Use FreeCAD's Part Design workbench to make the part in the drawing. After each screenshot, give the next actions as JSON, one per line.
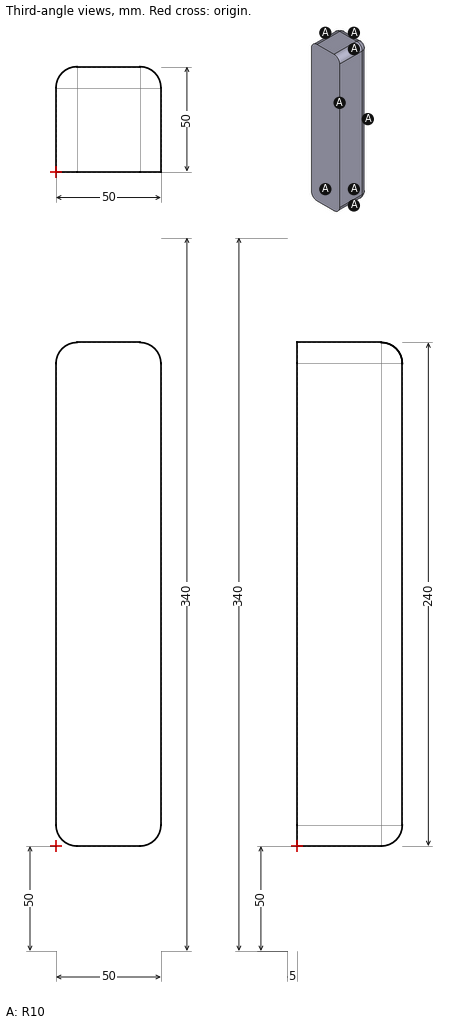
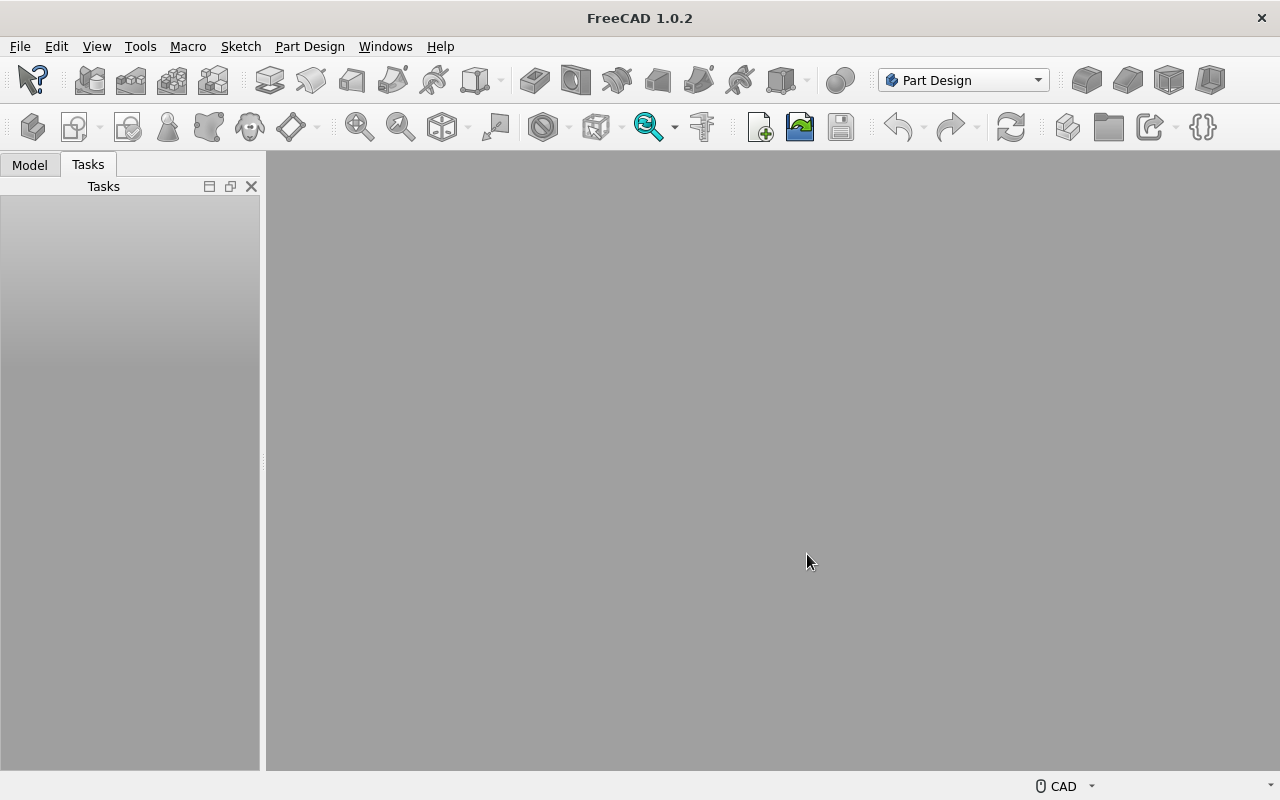
{"action": "key", "text": "ctrl+n"}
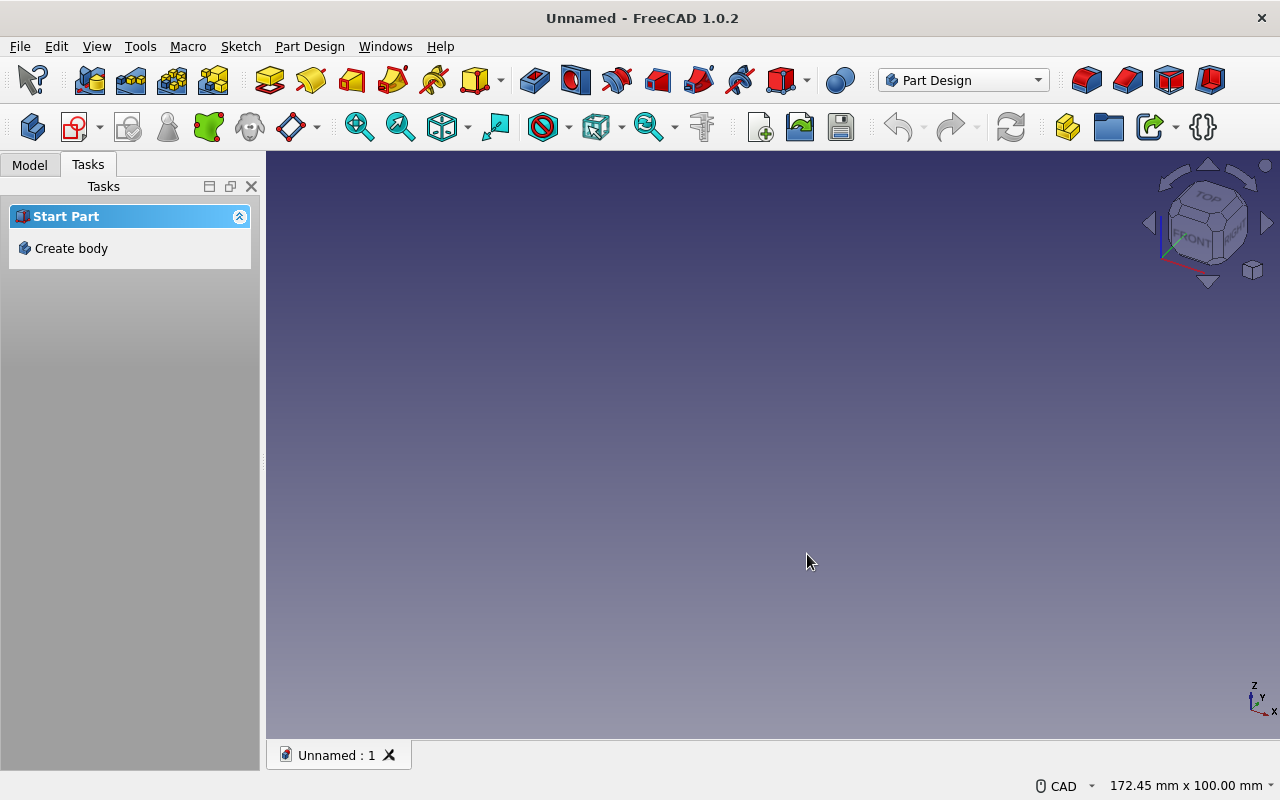
{"action": "left_click", "coordinate": [74, 128]}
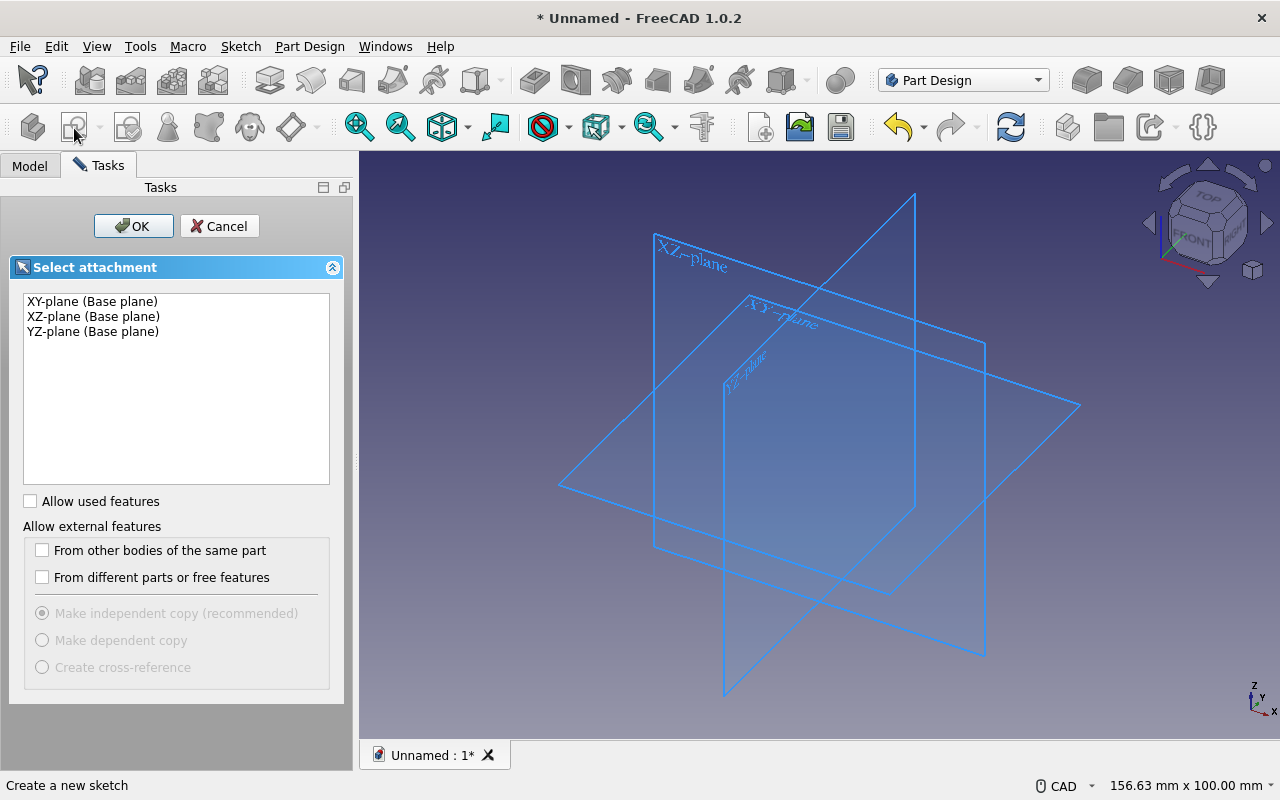
{"action": "left_click", "coordinate": [84, 302]}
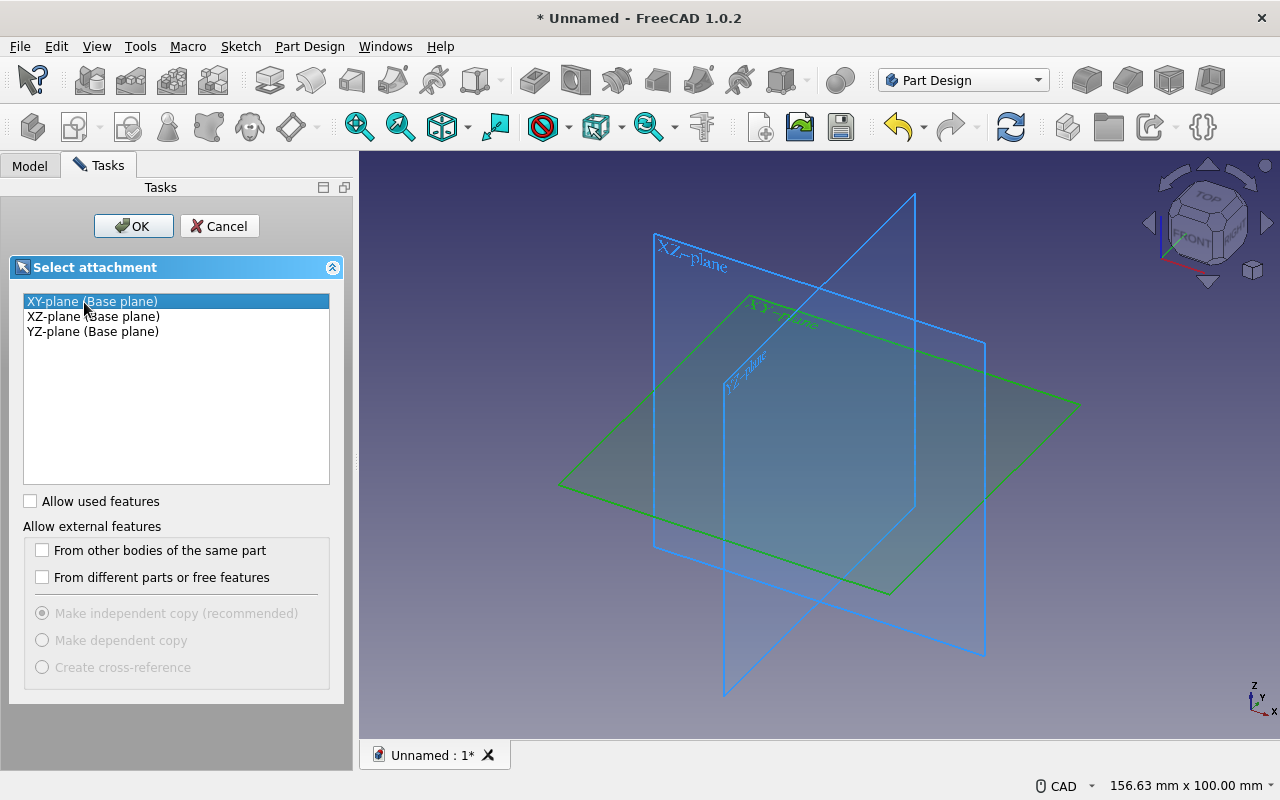
{"action": "left_click", "coordinate": [134, 226]}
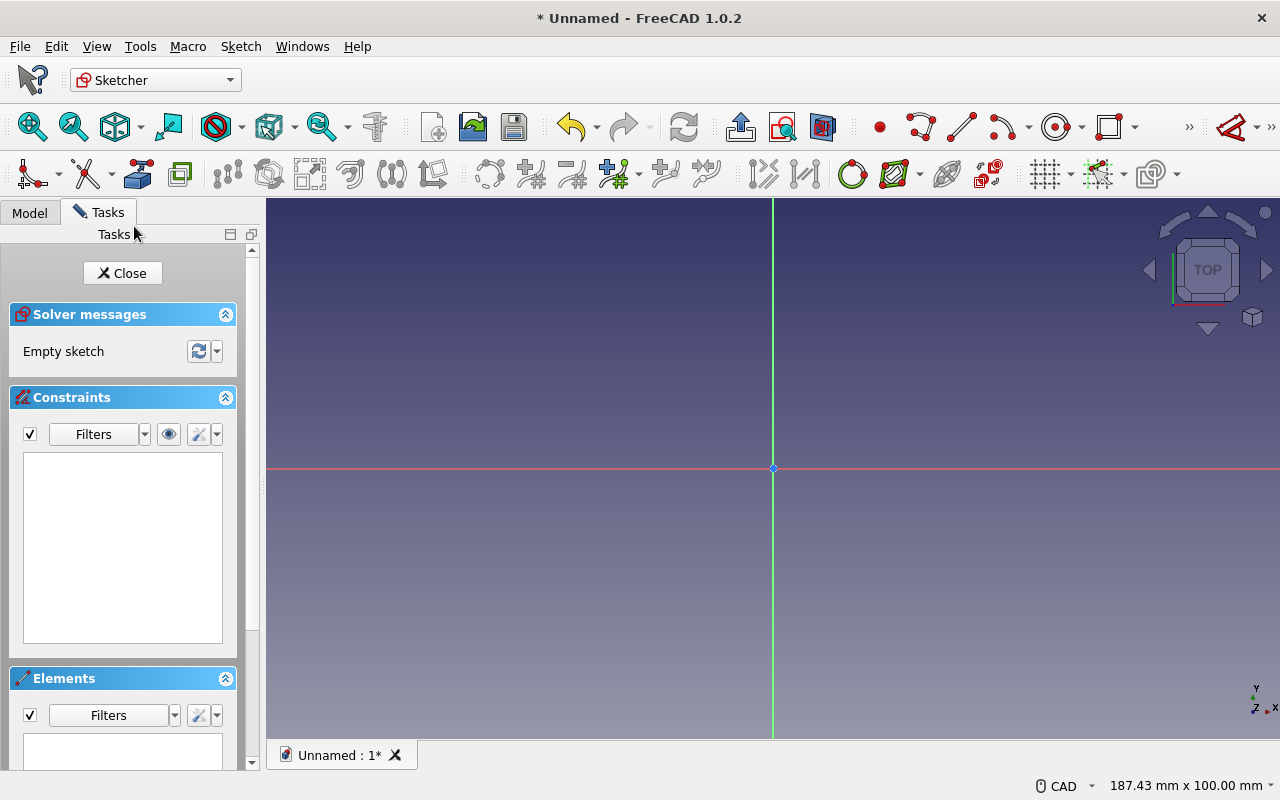
{"action": "scroll", "coordinate": [294, 711], "scroll_direction": "down", "scroll_amount": 1}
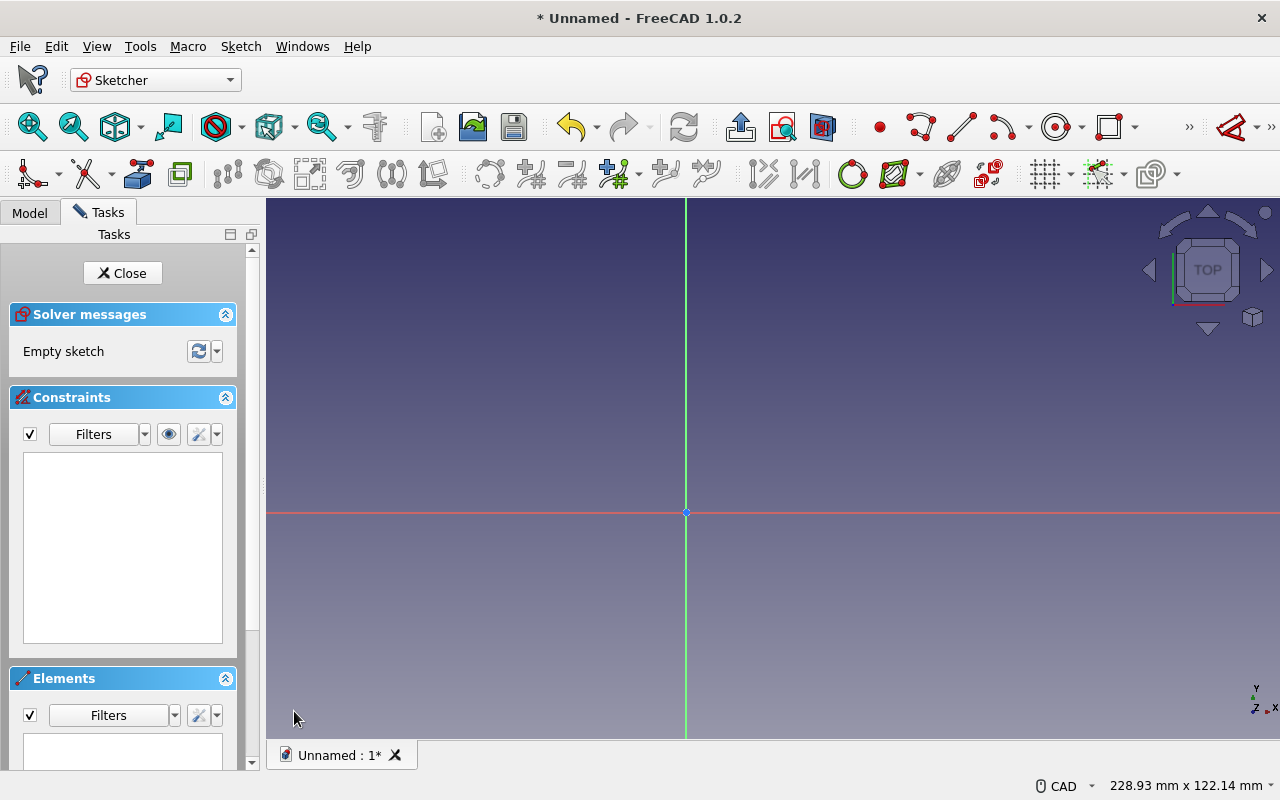
{"action": "scroll", "coordinate": [985, 266], "scroll_direction": "up", "scroll_amount": 2}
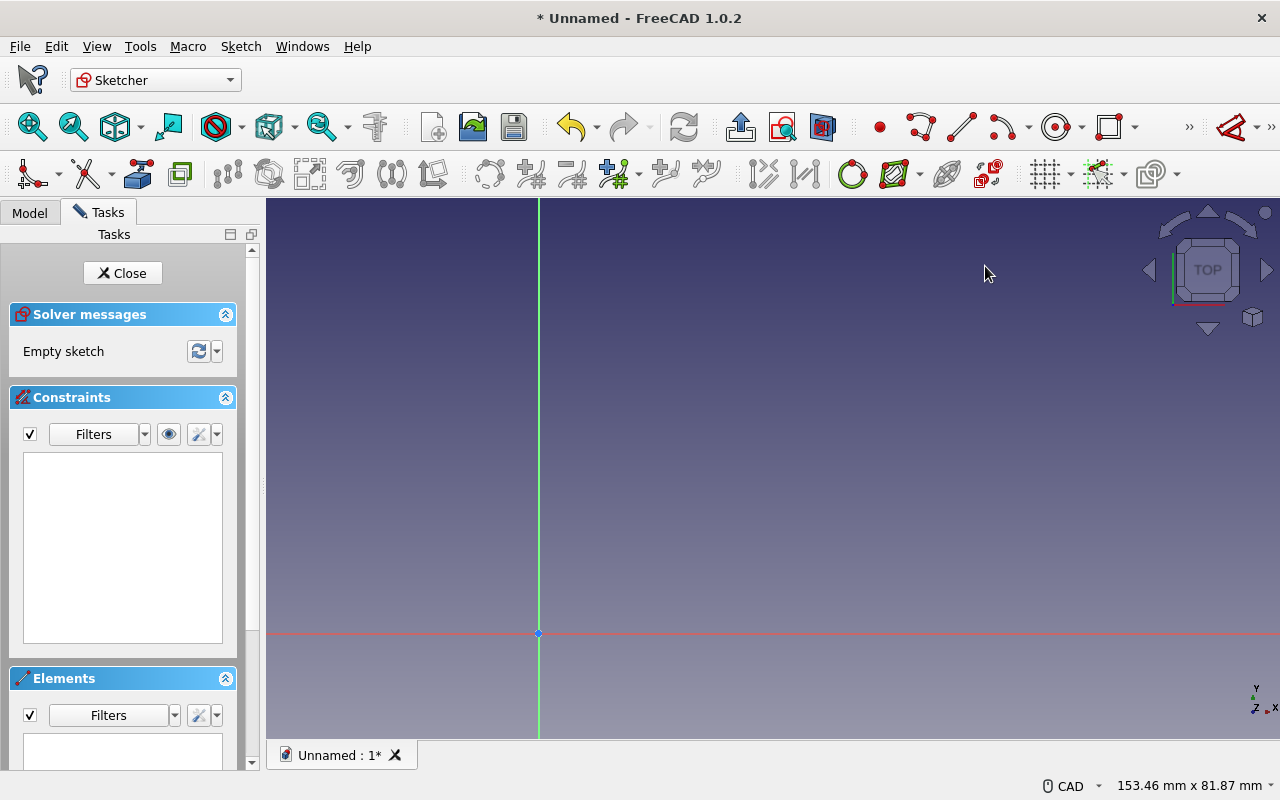
{"action": "key", "text": "g r"}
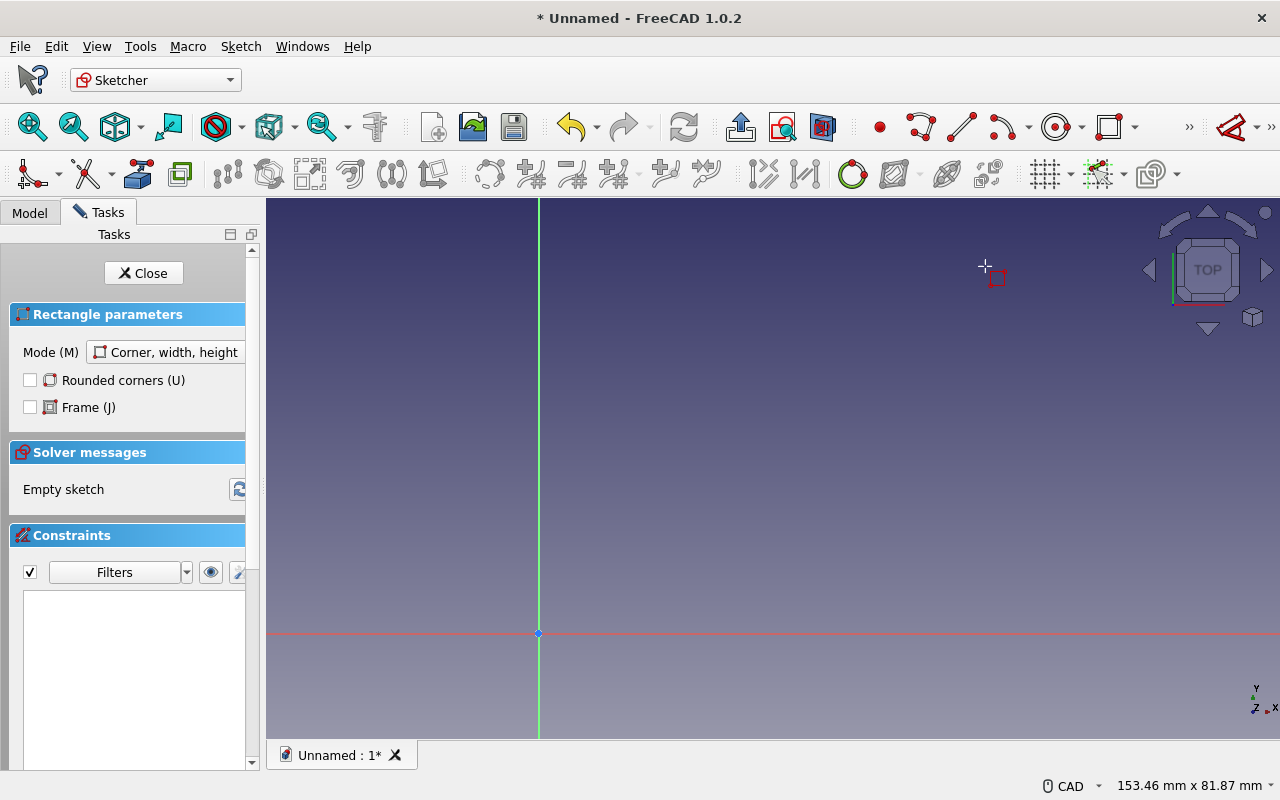
{"action": "left_click", "coordinate": [539, 634]}
{"action": "mouse_move", "coordinate": [869, 303]}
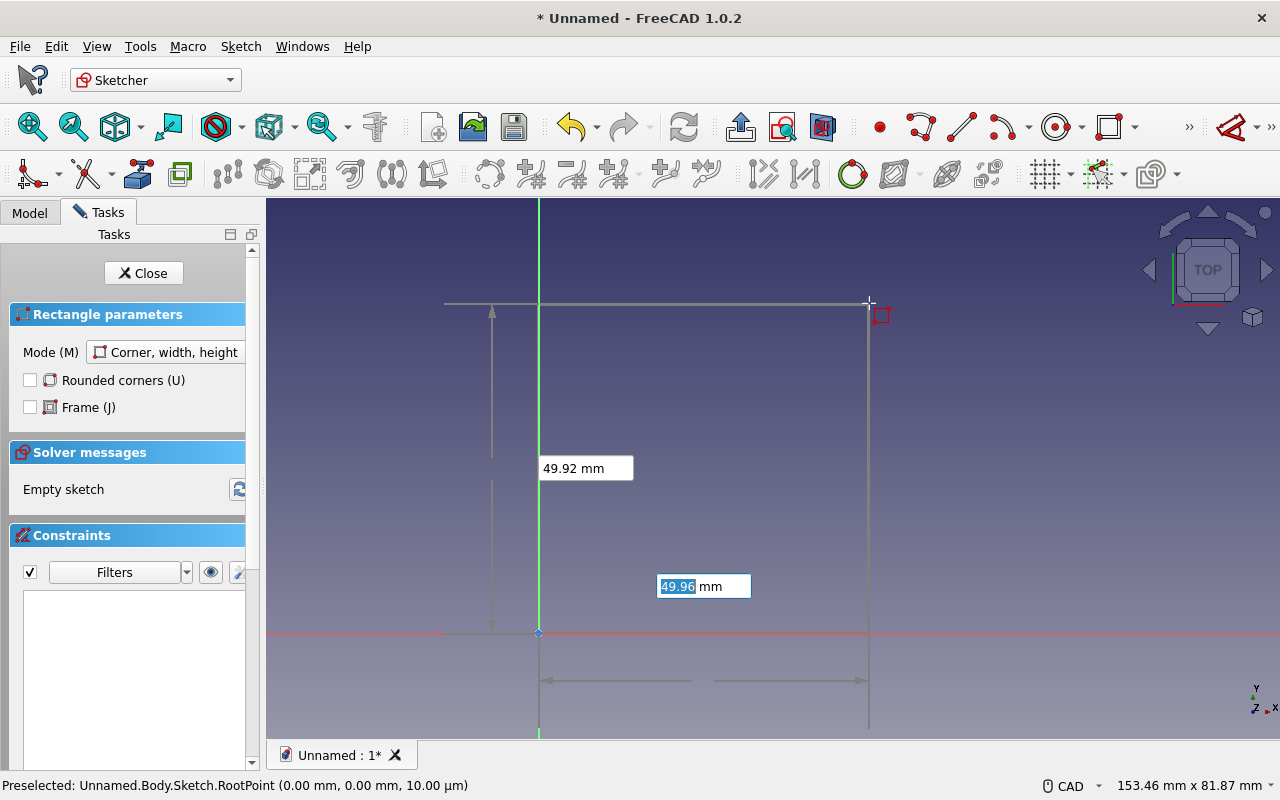
{"action": "type", "text": "50"}
{"action": "key", "text": "Tab"}
{"action": "type", "text": "50"}
{"action": "key", "text": "Return"}
{"action": "key", "text": "Escape"}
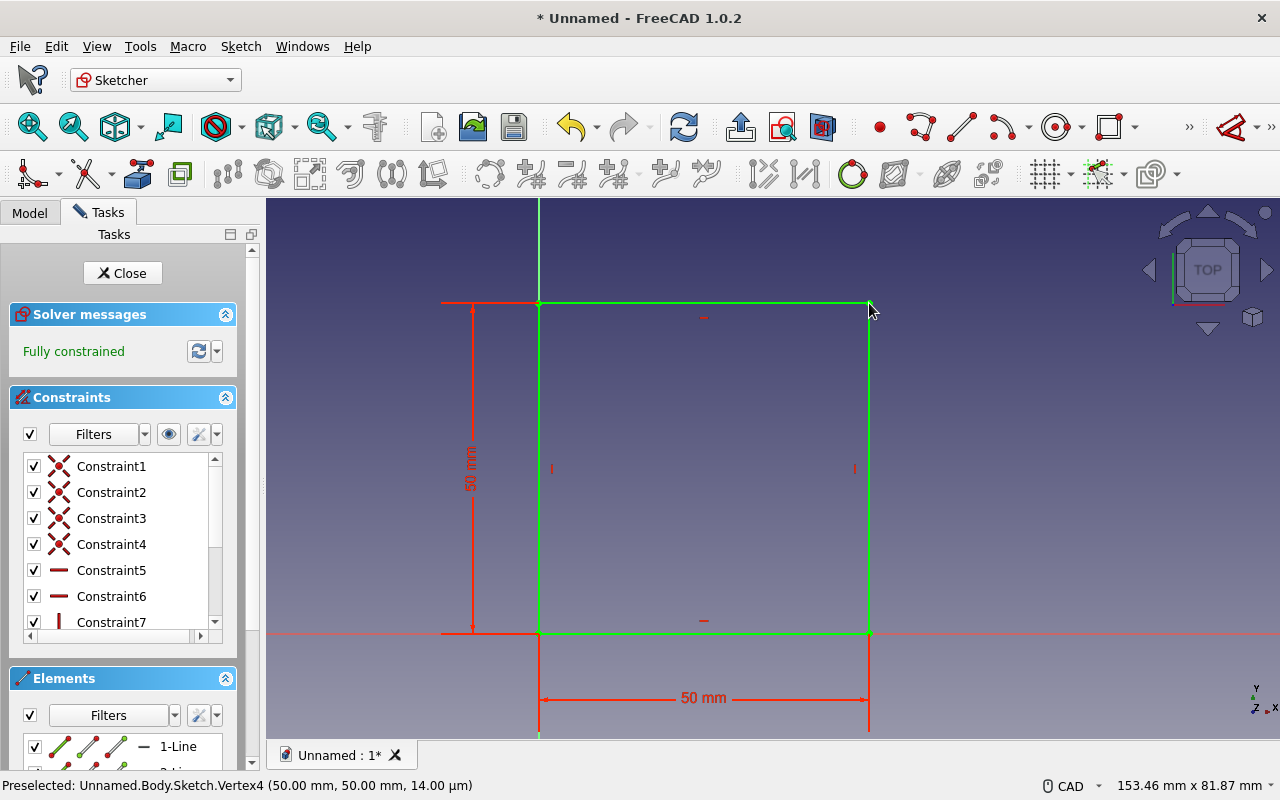
{"action": "left_click", "coordinate": [123, 273]}